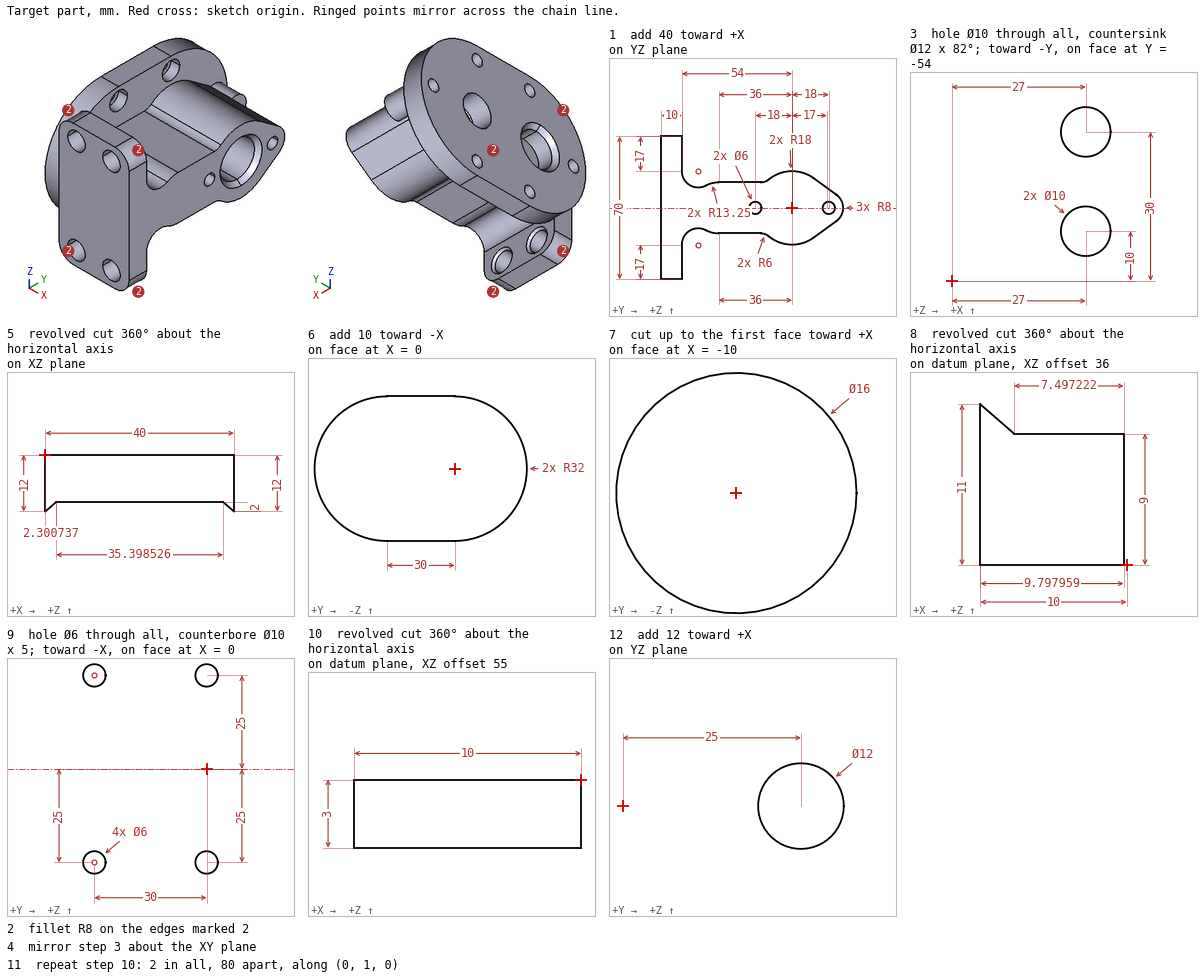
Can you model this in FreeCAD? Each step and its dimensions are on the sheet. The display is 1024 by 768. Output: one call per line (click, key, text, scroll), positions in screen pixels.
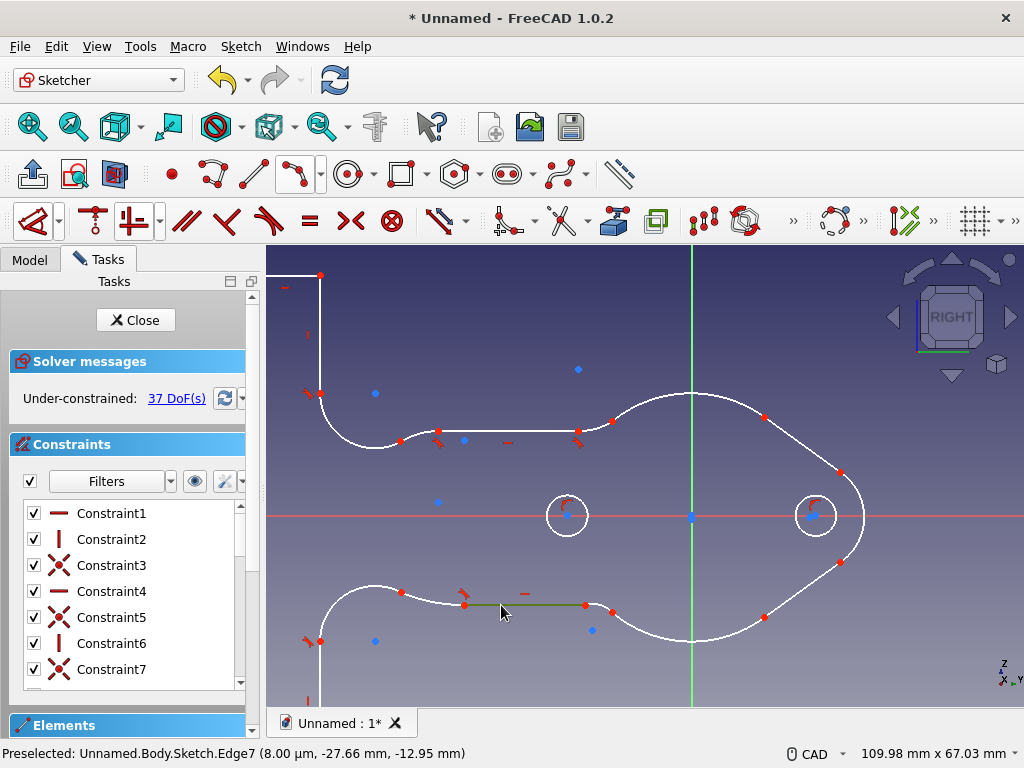
click(600, 605)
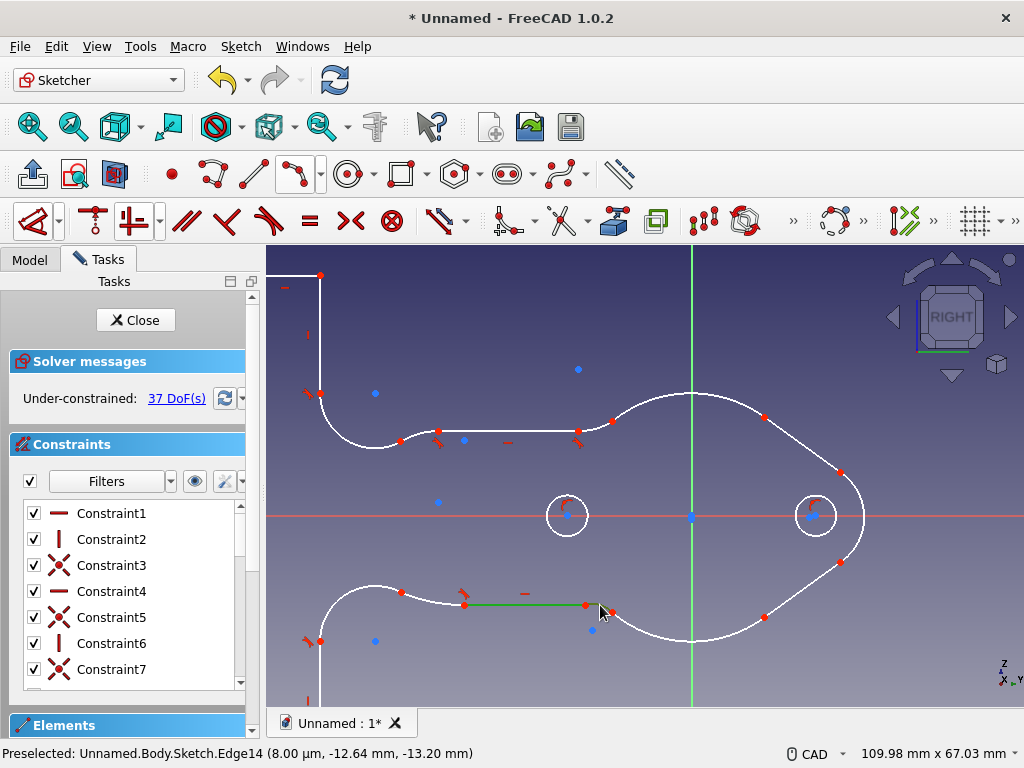
click(269, 222)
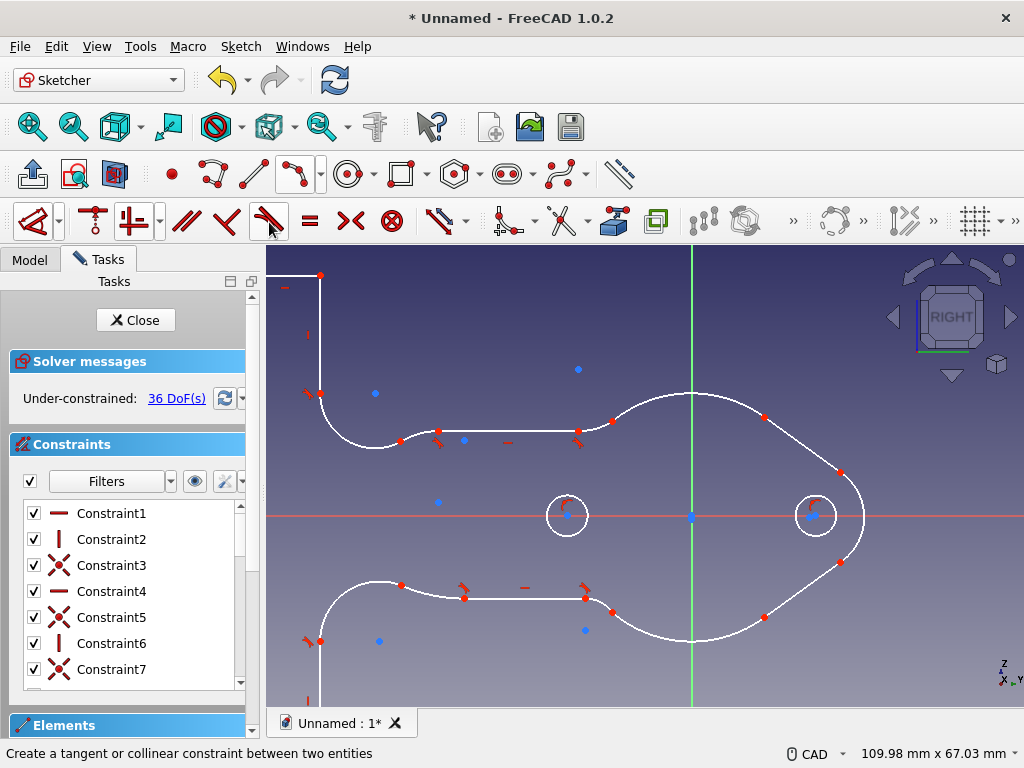
click(788, 601)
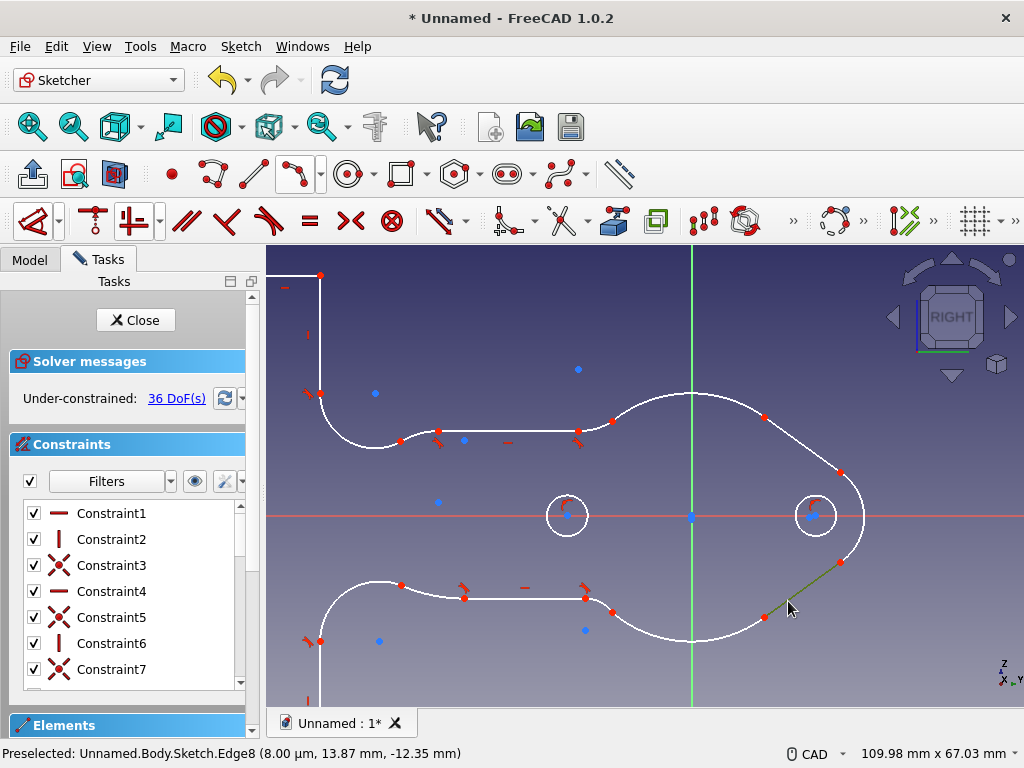
click(655, 636)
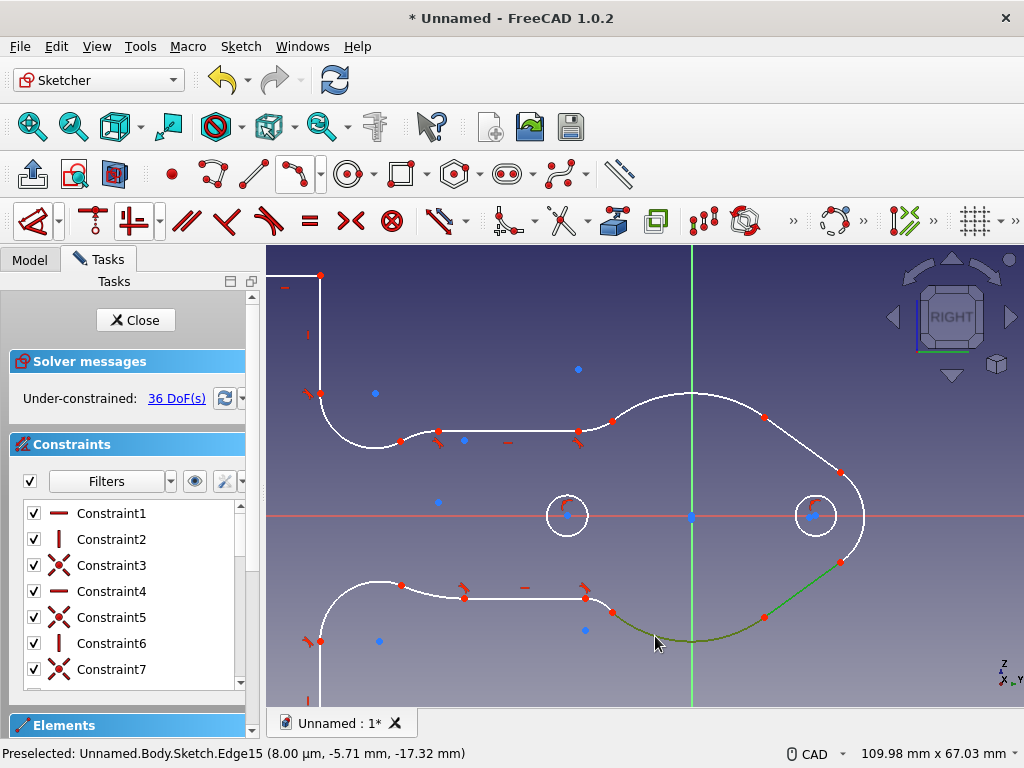
click(269, 222)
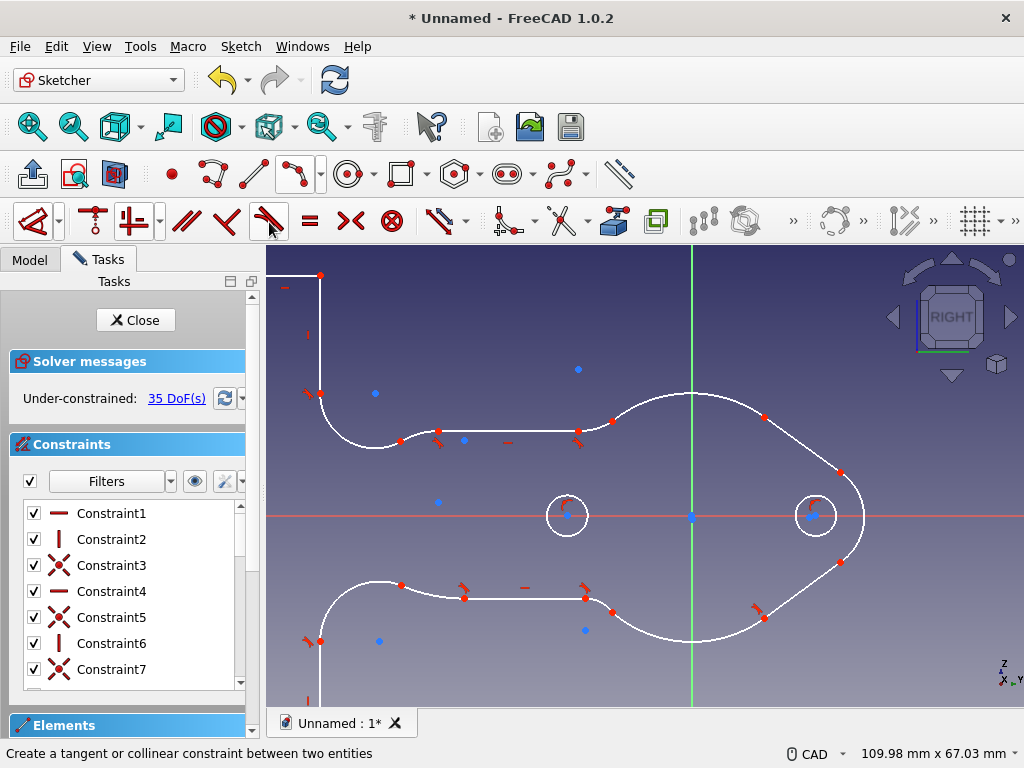
click(788, 601)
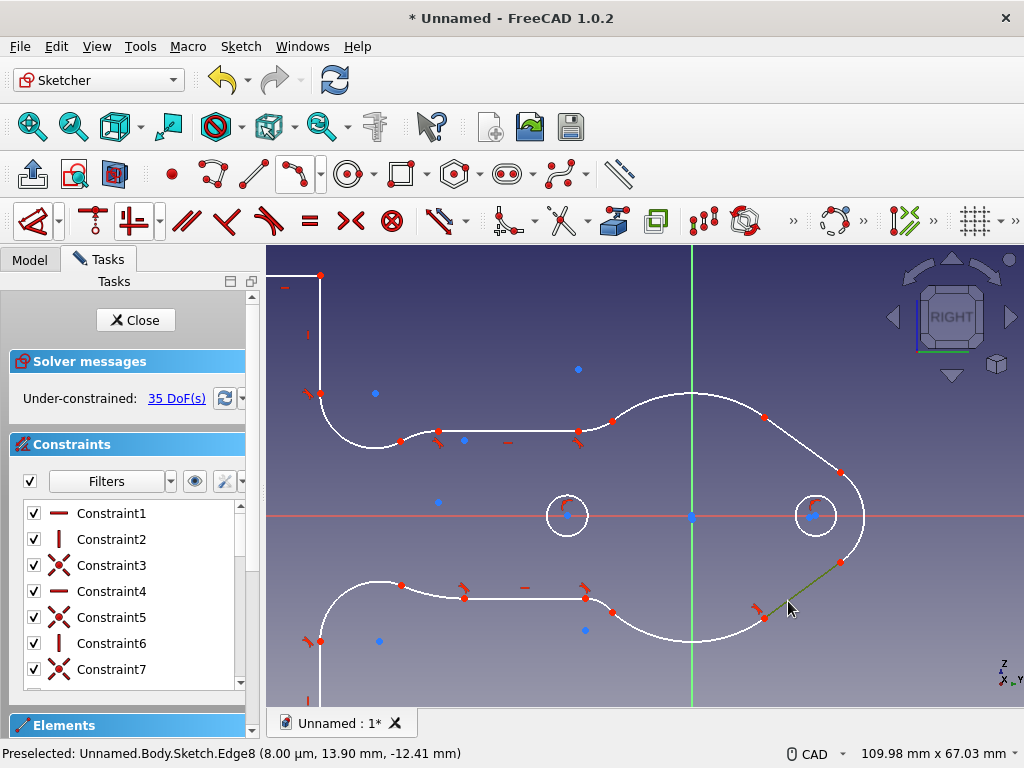
click(855, 547)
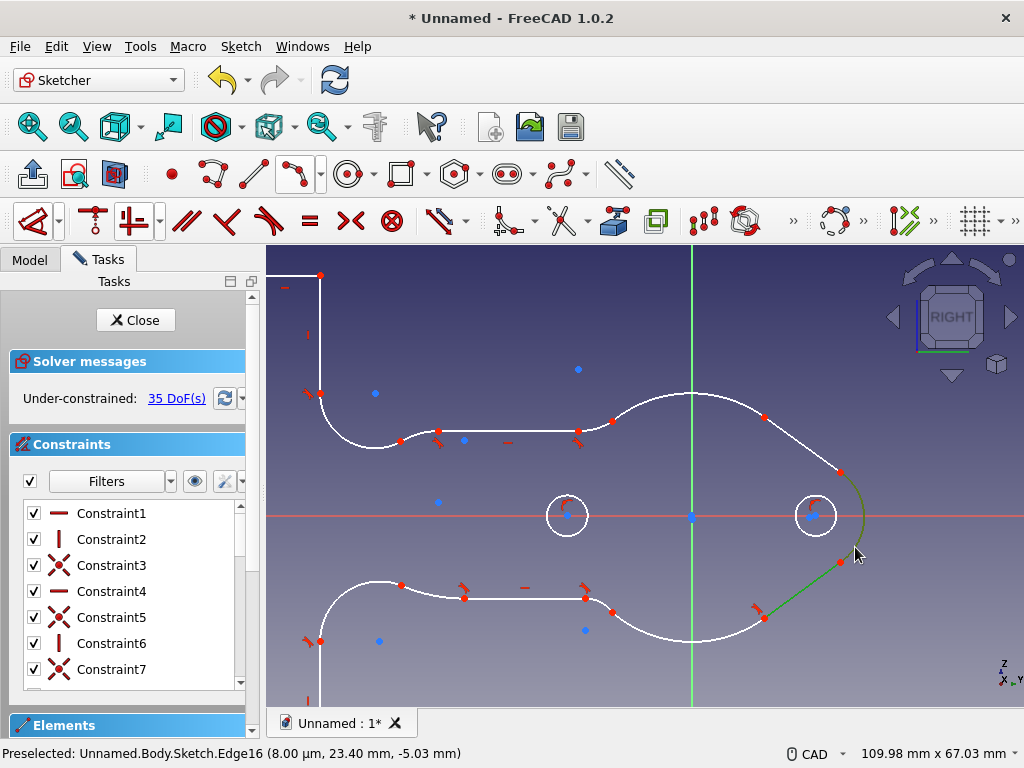
click(269, 222)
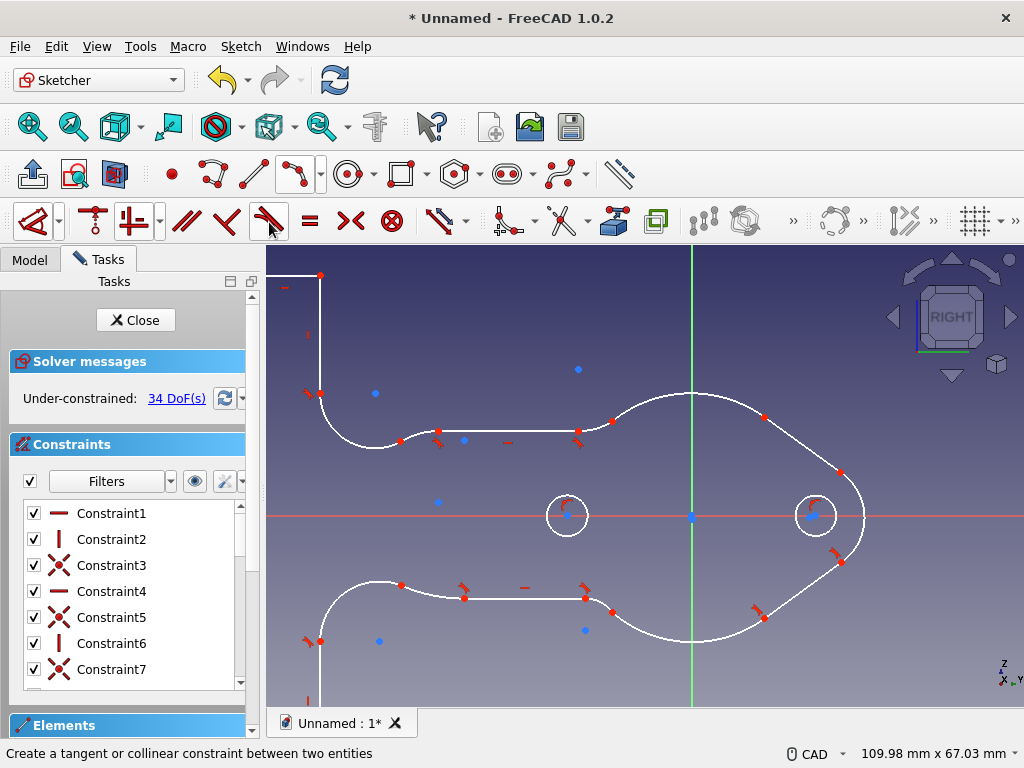
click(818, 456)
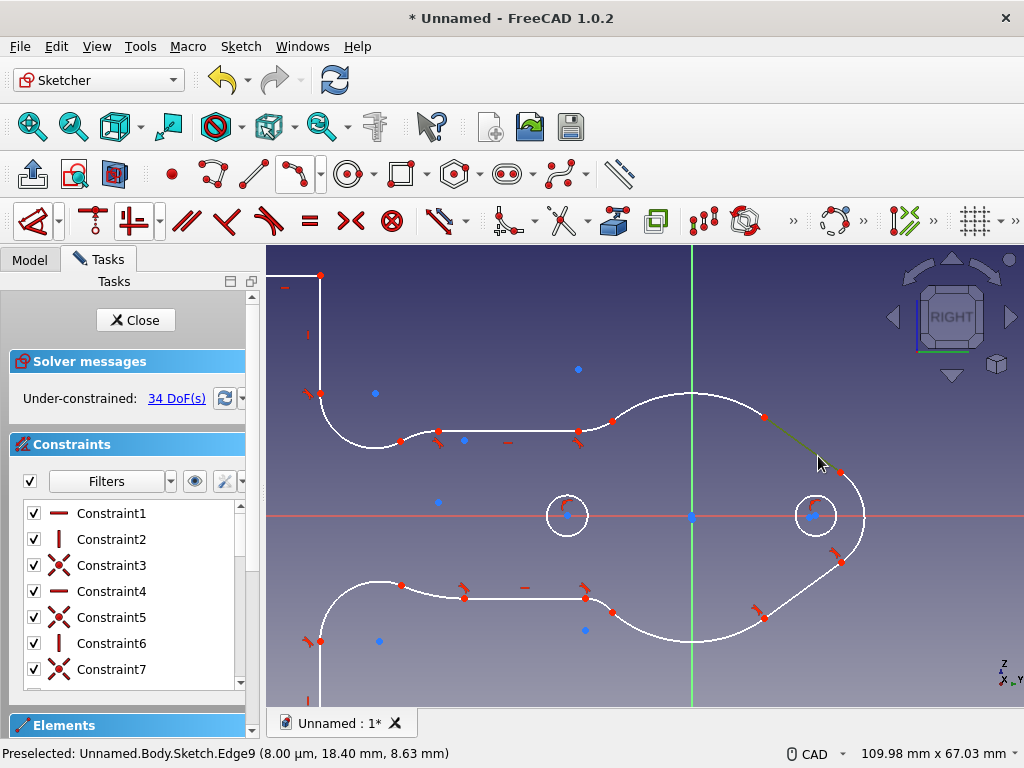
click(856, 547)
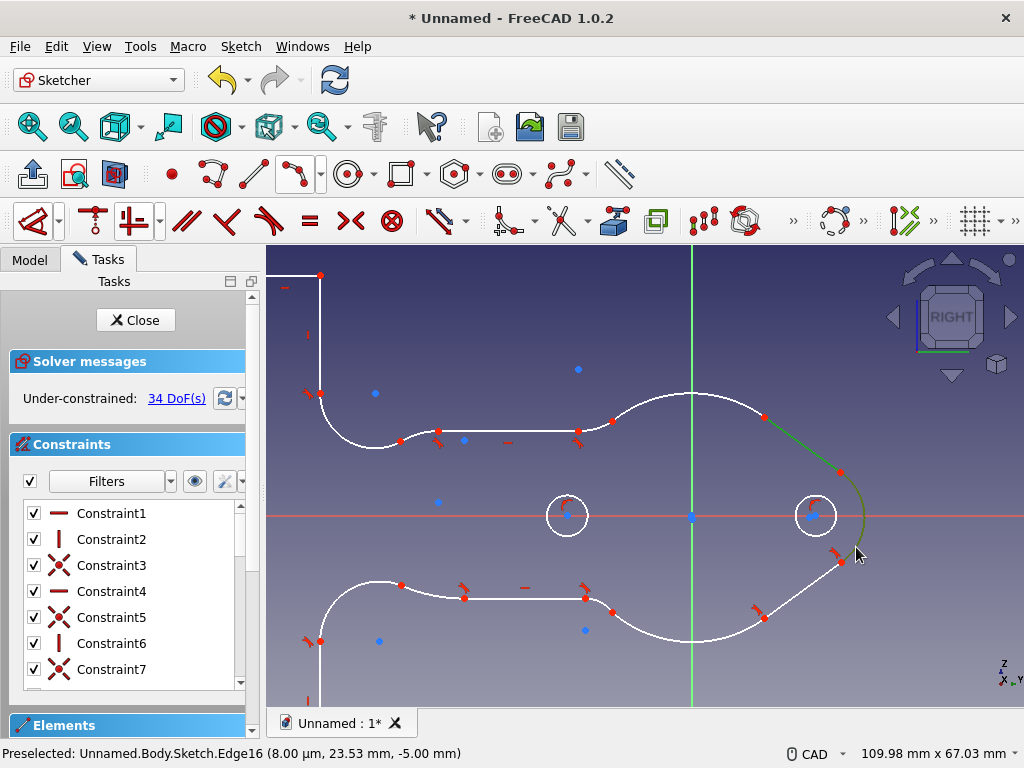
click(269, 222)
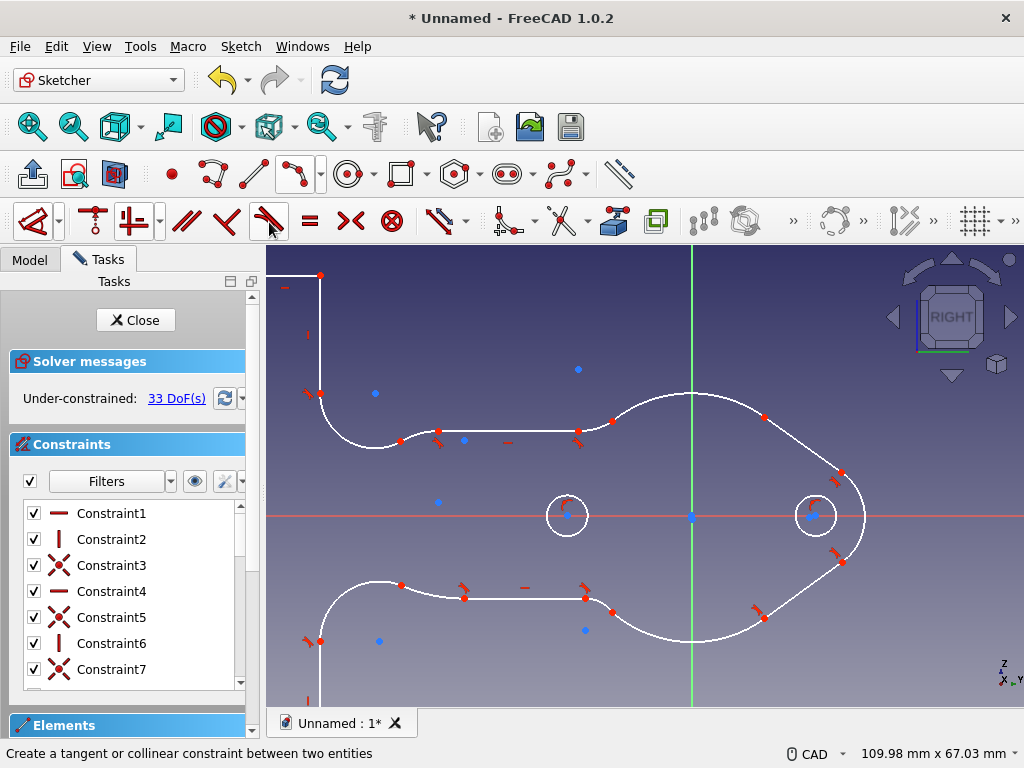
click(819, 456)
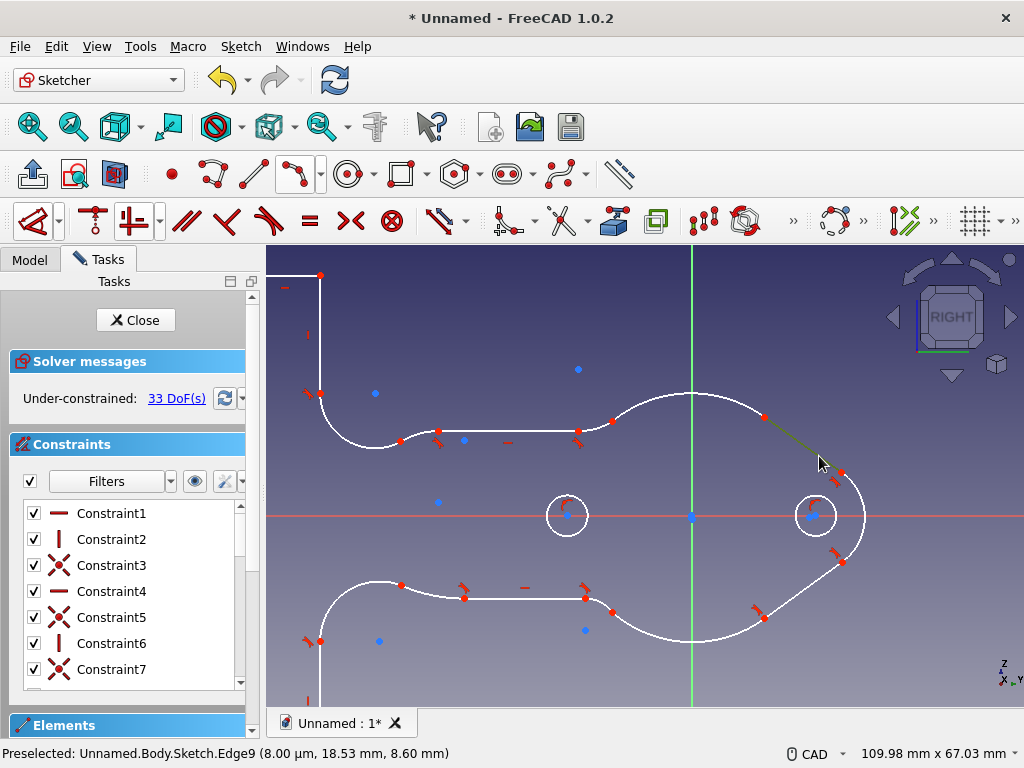
click(720, 397)